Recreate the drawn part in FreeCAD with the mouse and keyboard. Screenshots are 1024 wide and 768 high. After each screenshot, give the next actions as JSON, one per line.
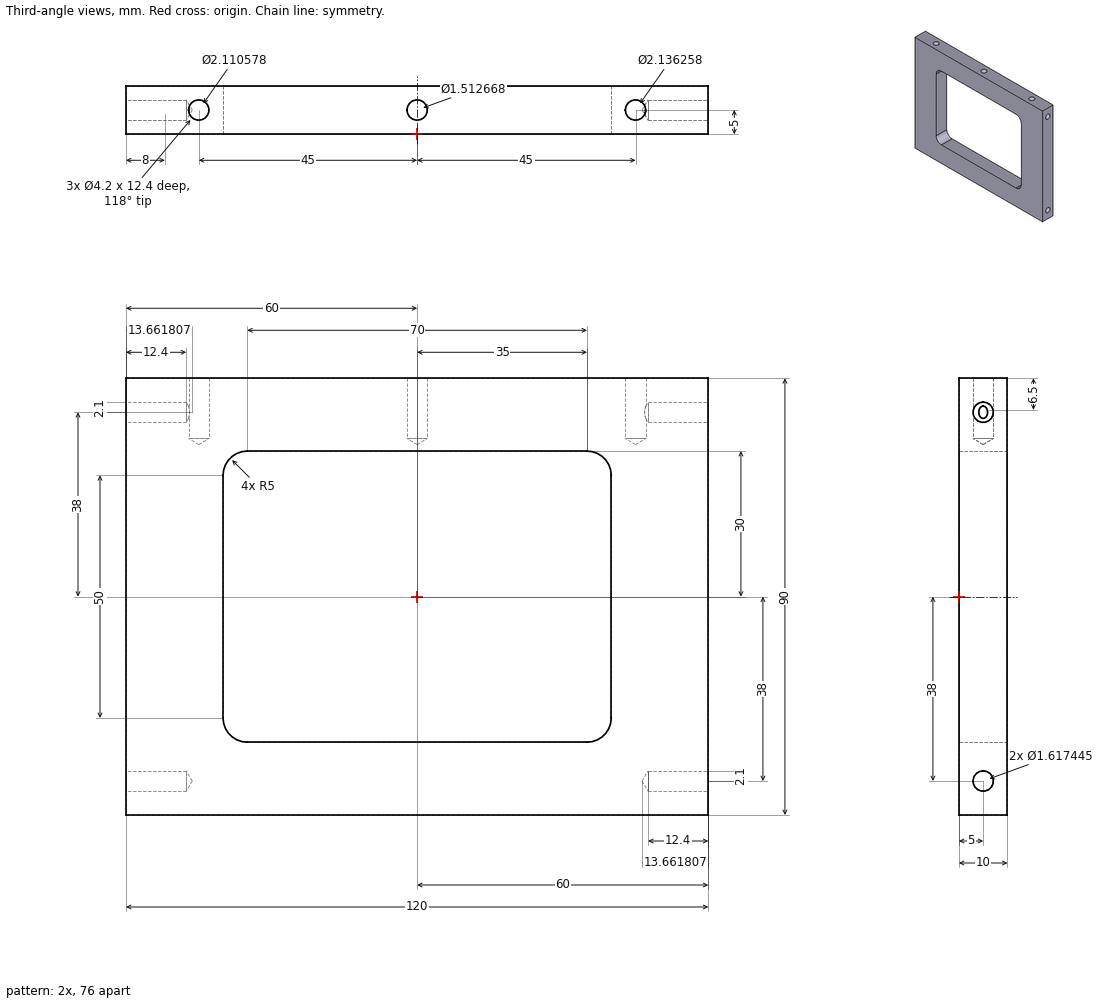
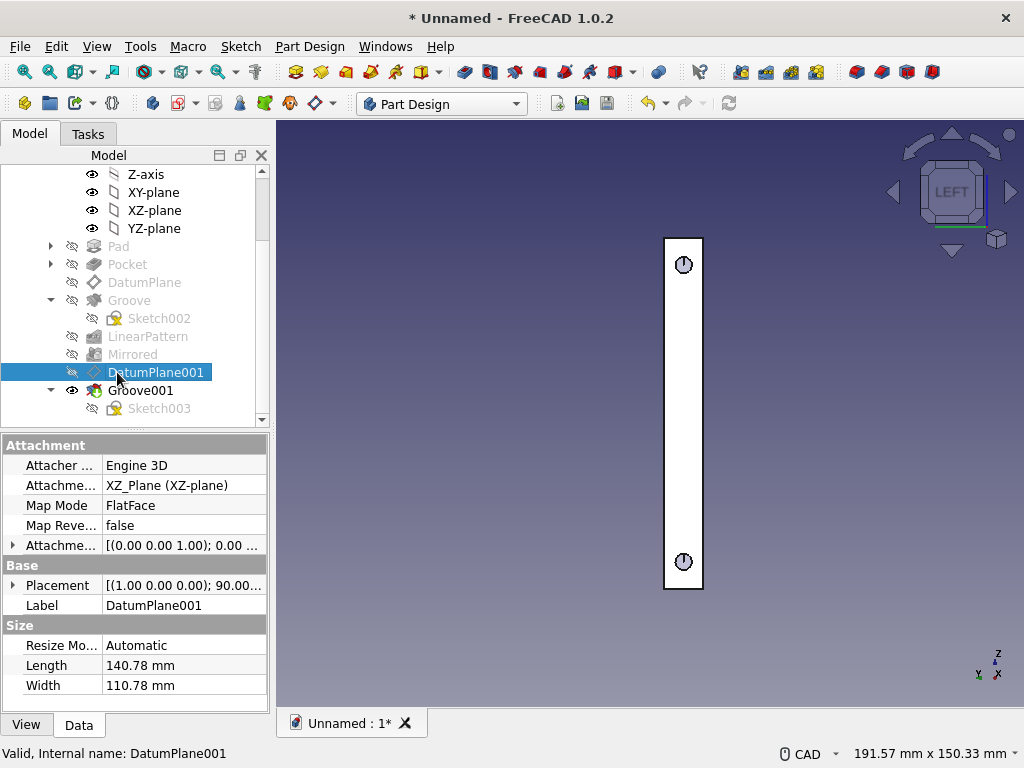
{"action": "key", "text": "0"}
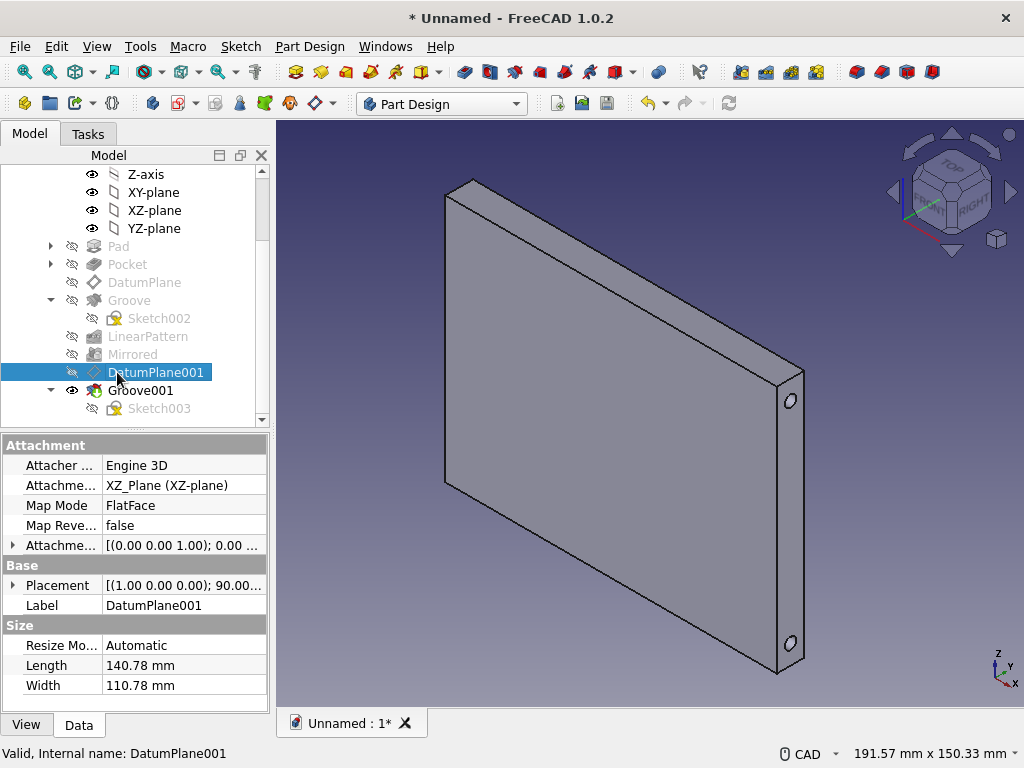
{"action": "left_click", "coordinate": [767, 364]}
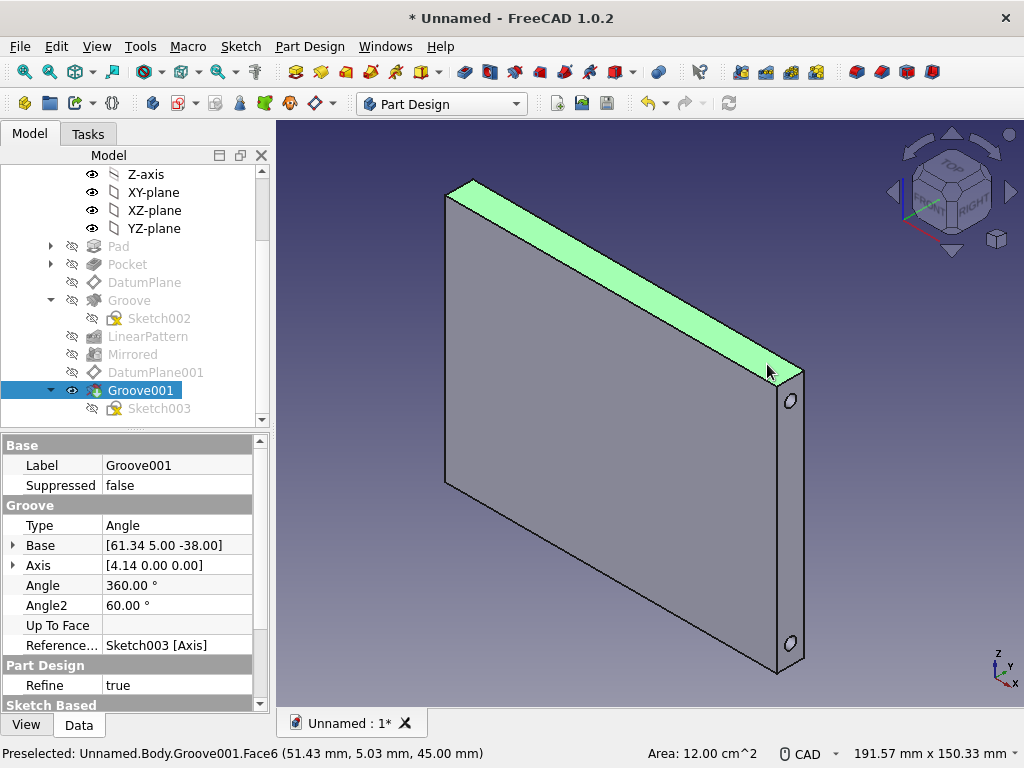
{"action": "left_click", "coordinate": [178, 104]}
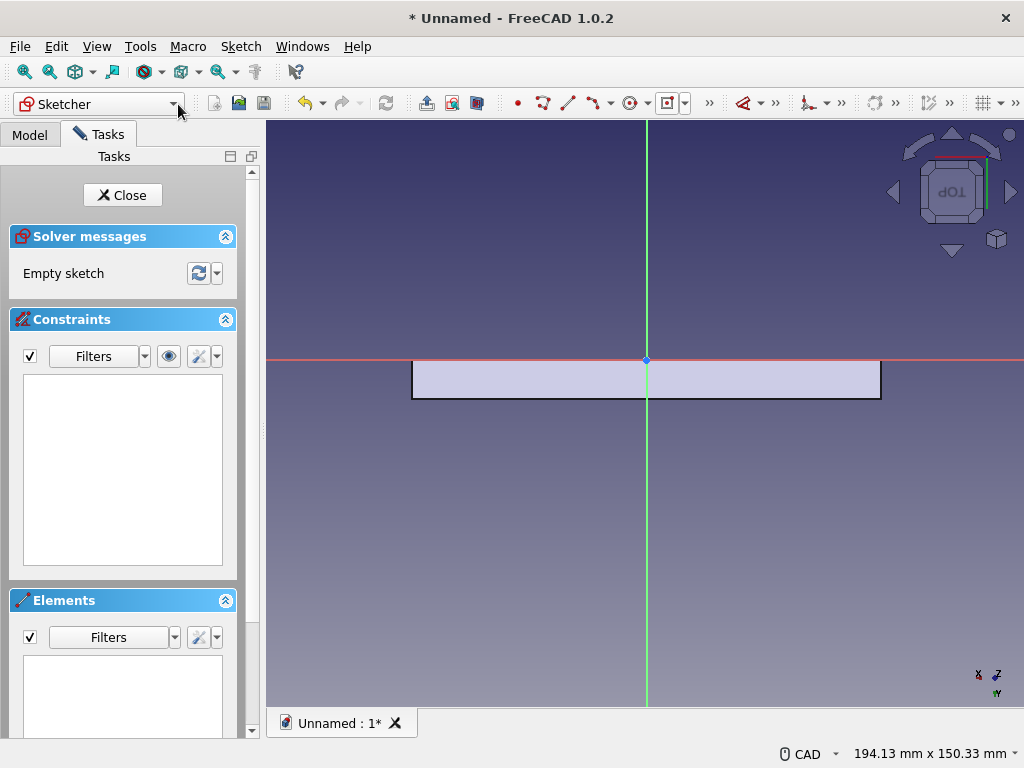
{"action": "left_click", "coordinate": [630, 104]}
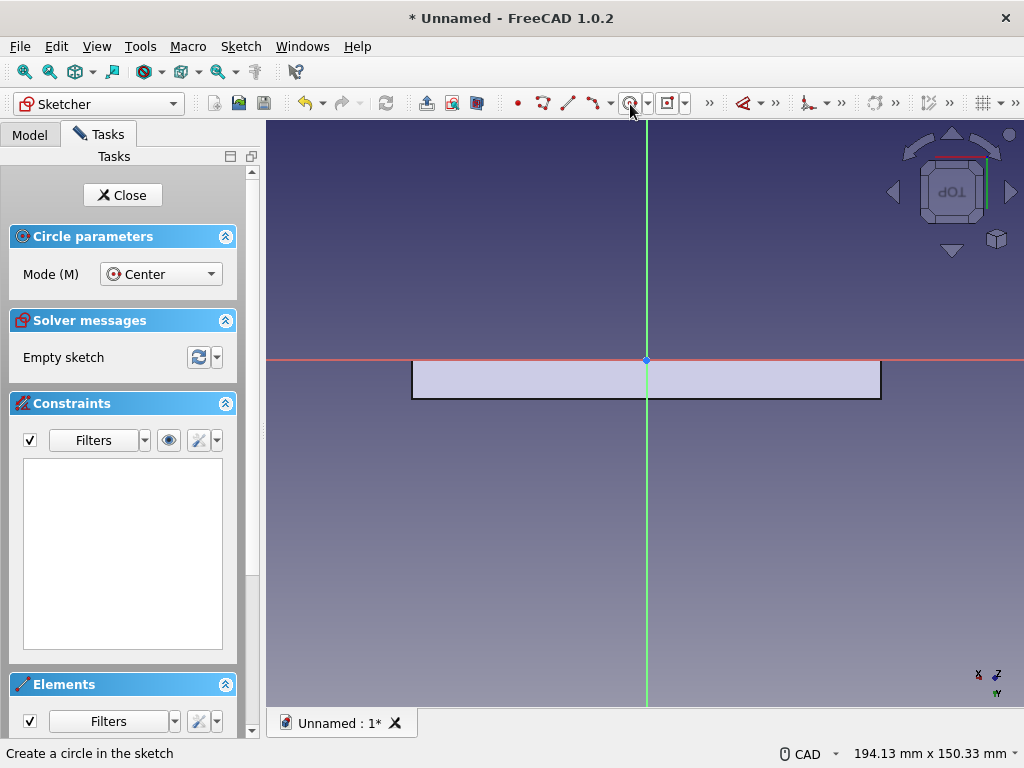
{"action": "scroll", "coordinate": [471, 380], "scroll_direction": "up", "scroll_amount": 9}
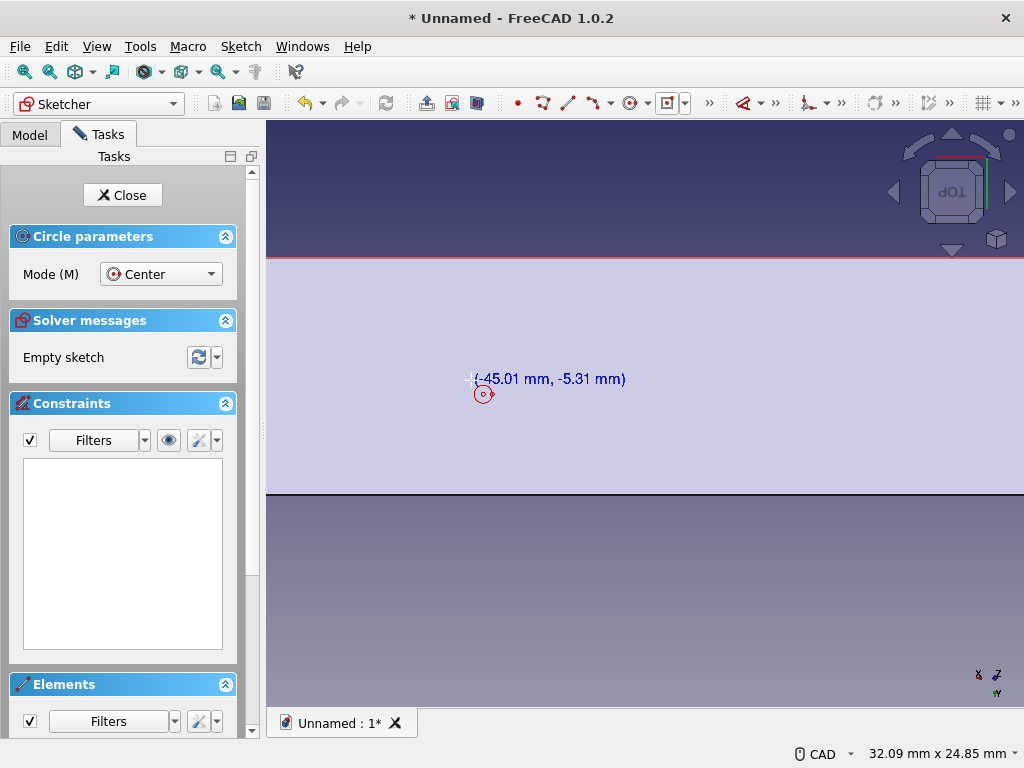
{"action": "scroll", "coordinate": [335, 435], "scroll_direction": "down", "scroll_amount": 8}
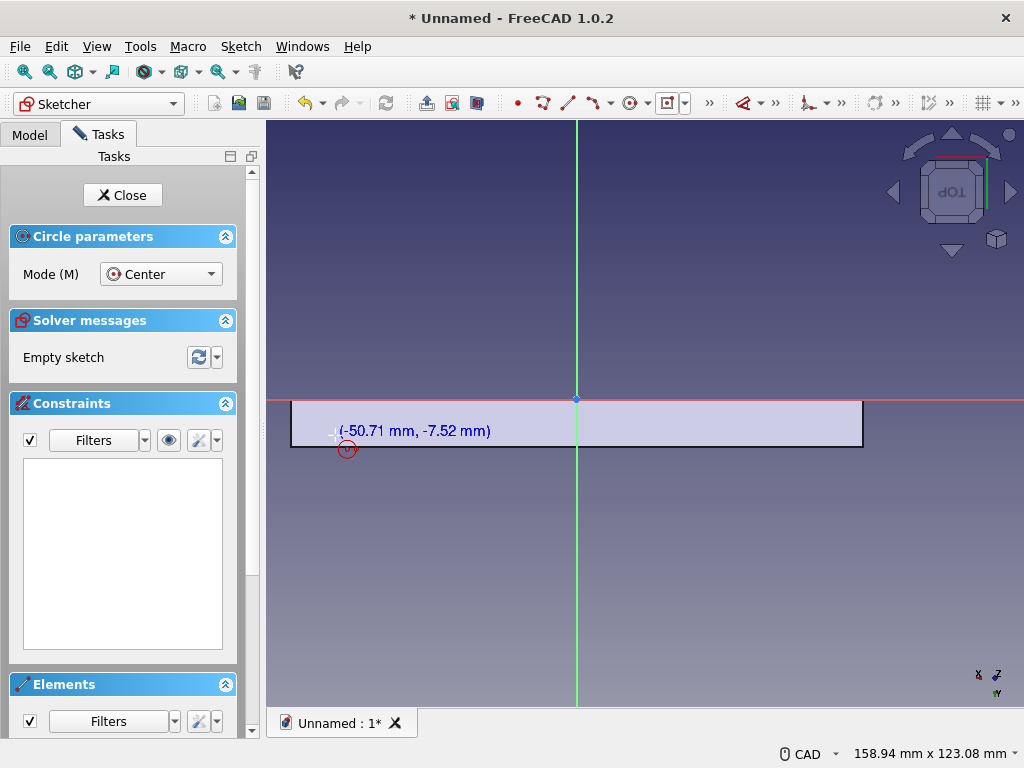
{"action": "left_click", "coordinate": [362, 424]}
{"action": "mouse_move", "coordinate": [366, 420]}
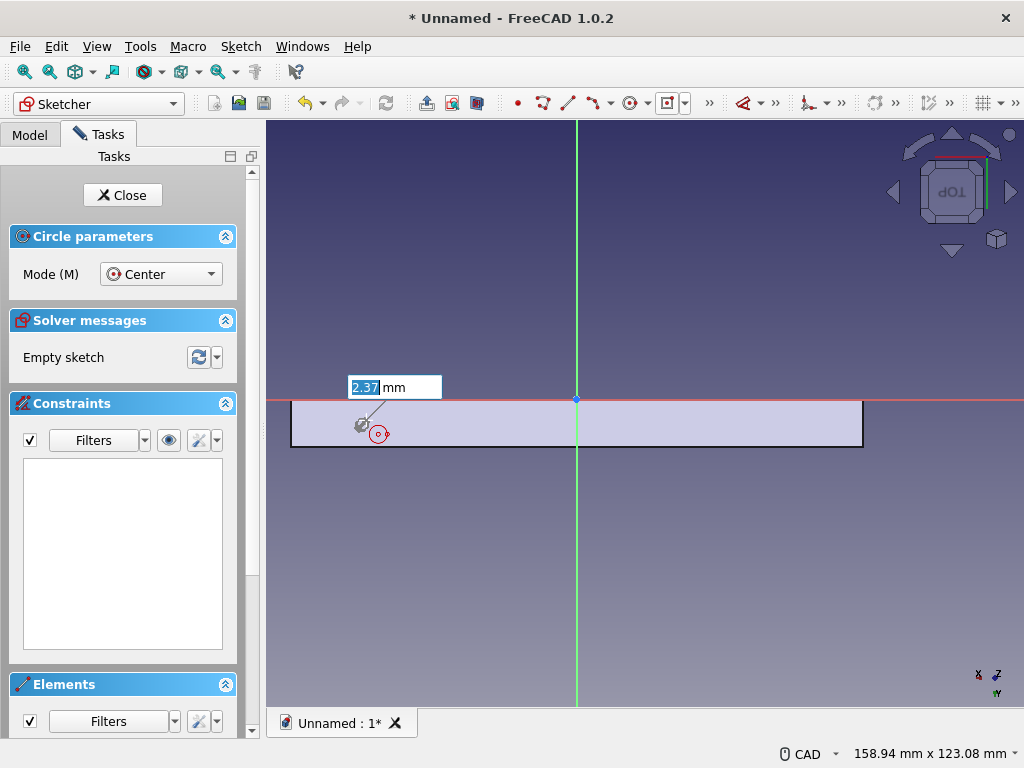
{"action": "type", "text": "2.136258"}
{"action": "key", "text": "Return"}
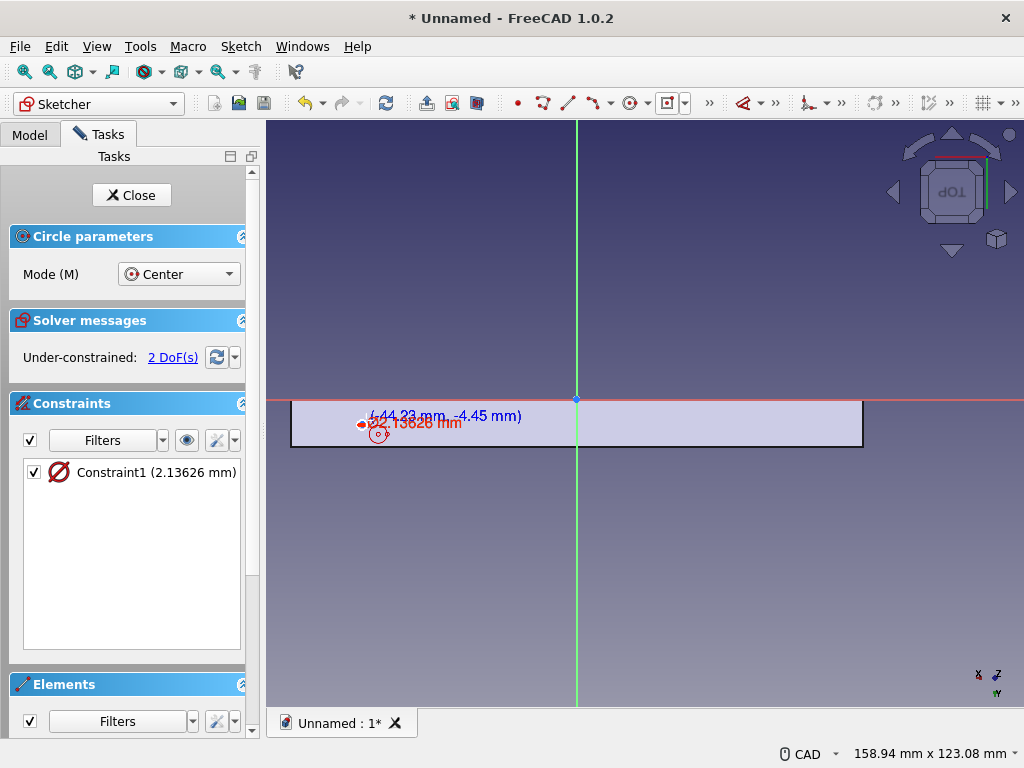
{"action": "scroll", "coordinate": [577, 424], "scroll_direction": "up", "scroll_amount": 10}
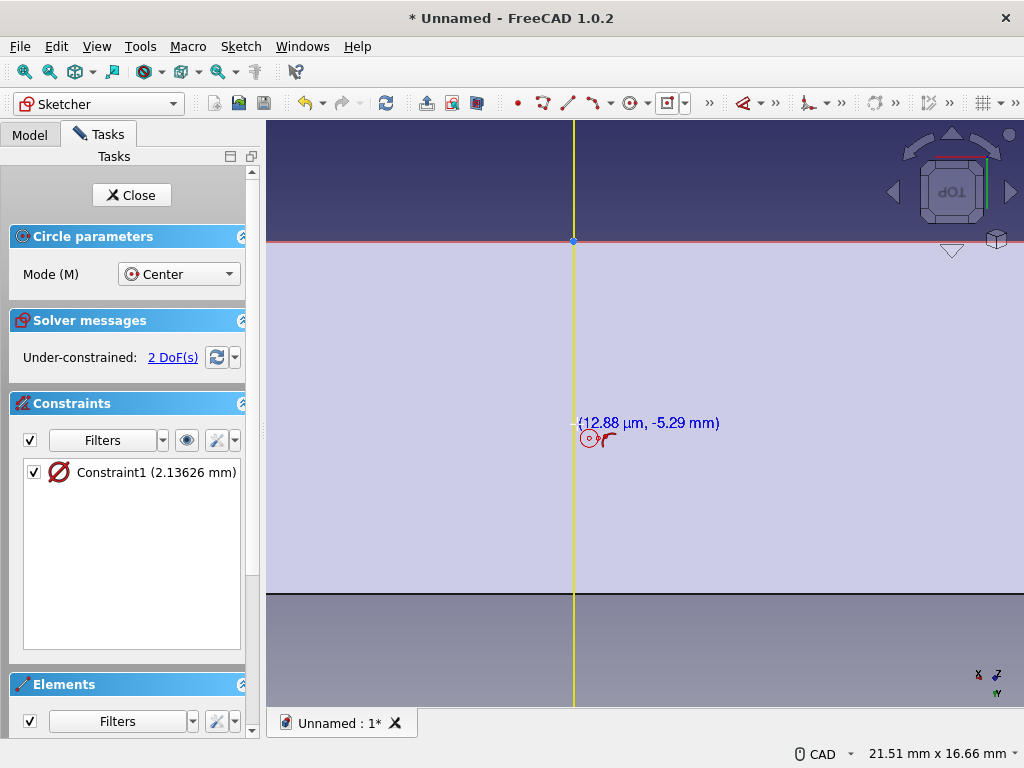
{"action": "scroll", "coordinate": [577, 424], "scroll_direction": "down", "scroll_amount": 10}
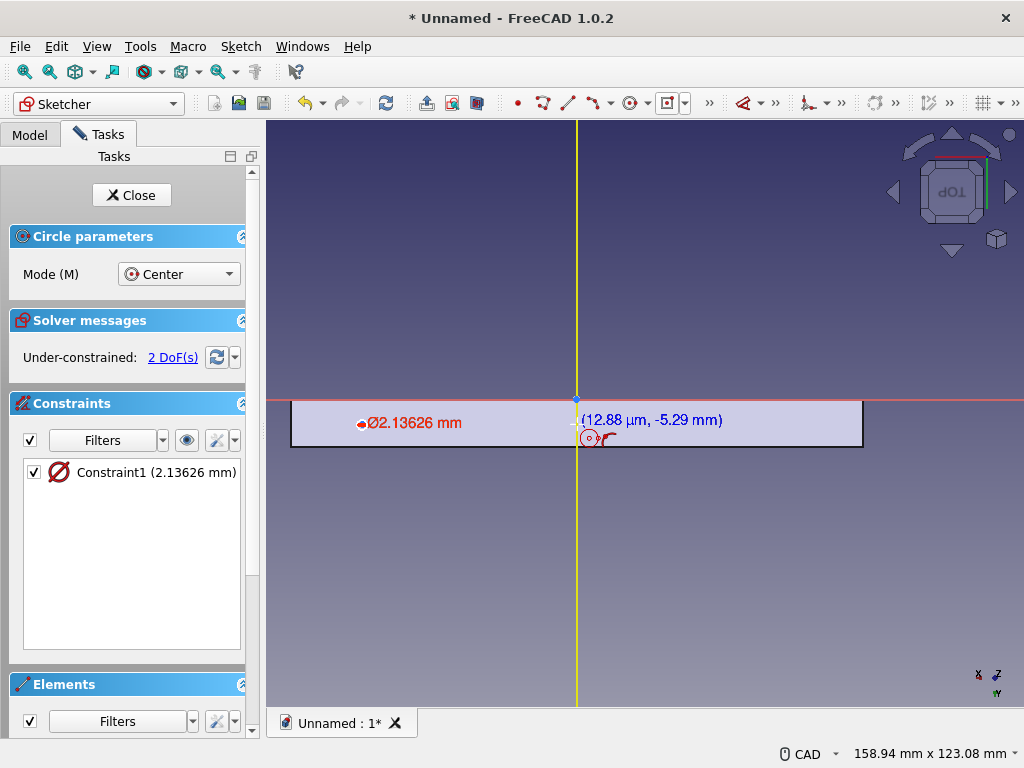
{"action": "left_click", "coordinate": [577, 424]}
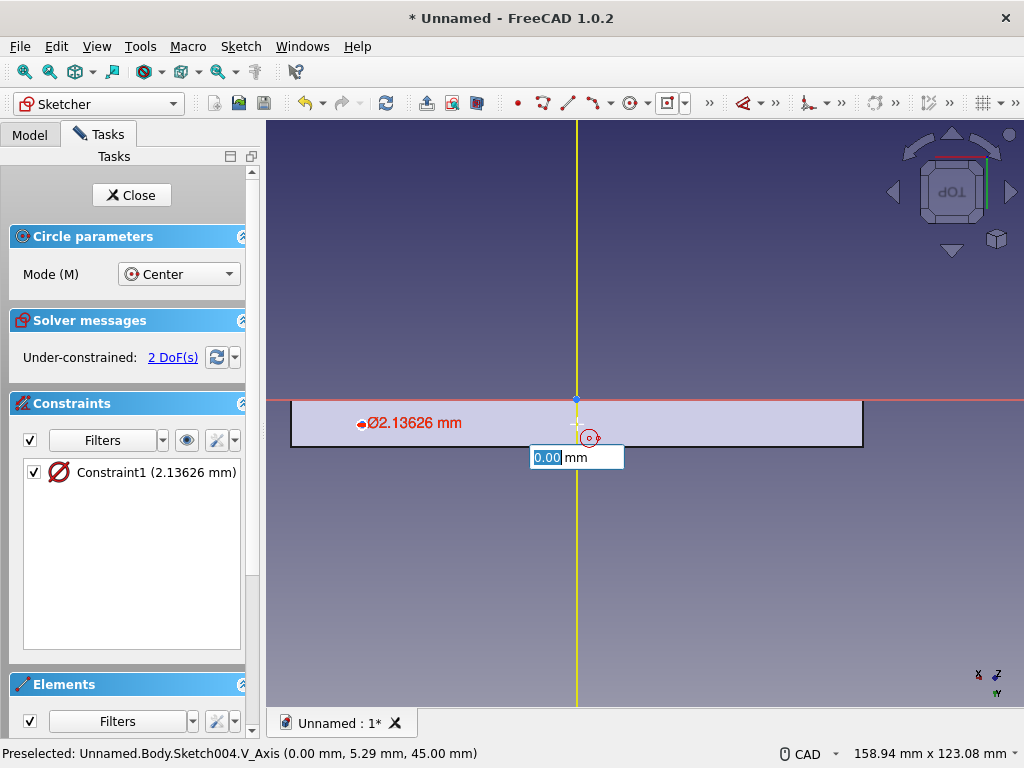
{"action": "scroll", "coordinate": [580, 422], "scroll_direction": "up", "scroll_amount": 8}
{"action": "mouse_move", "coordinate": [580, 422]}